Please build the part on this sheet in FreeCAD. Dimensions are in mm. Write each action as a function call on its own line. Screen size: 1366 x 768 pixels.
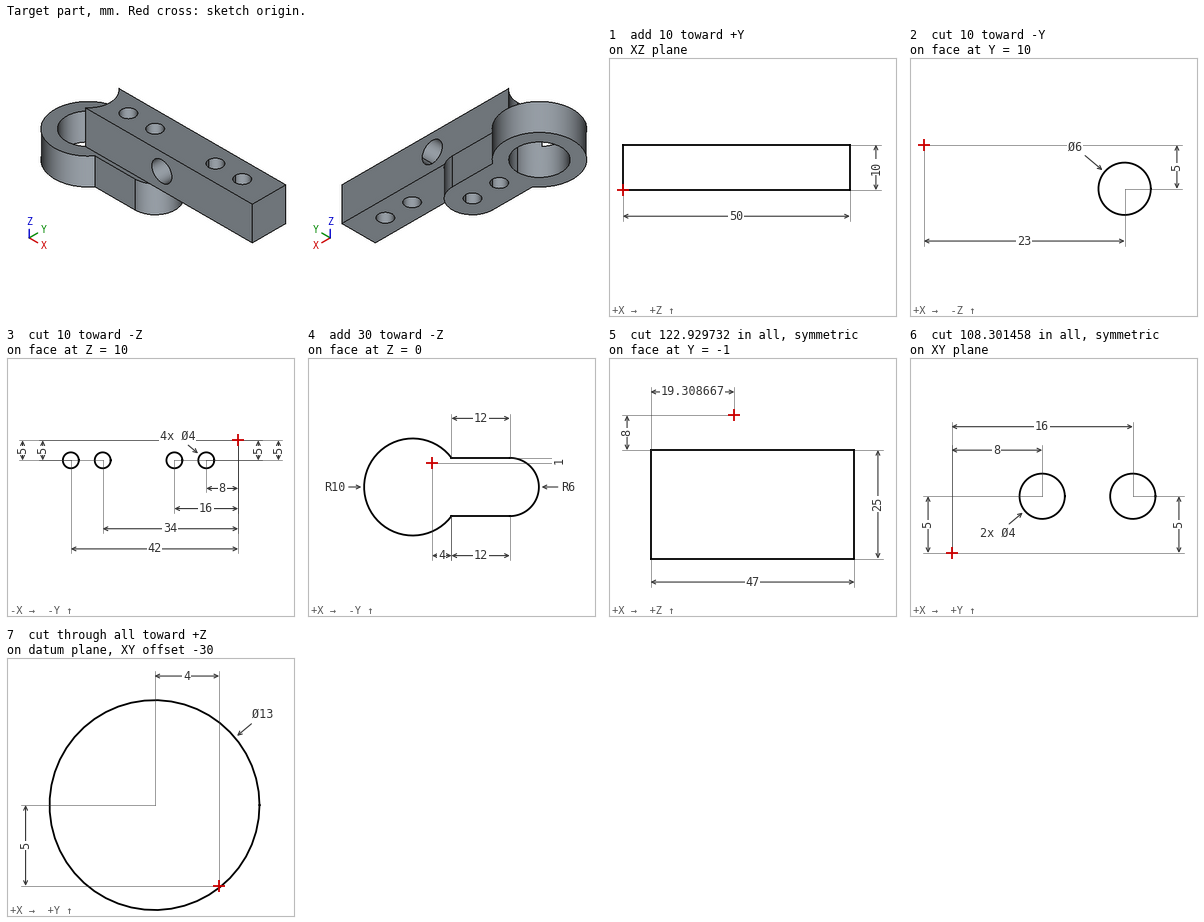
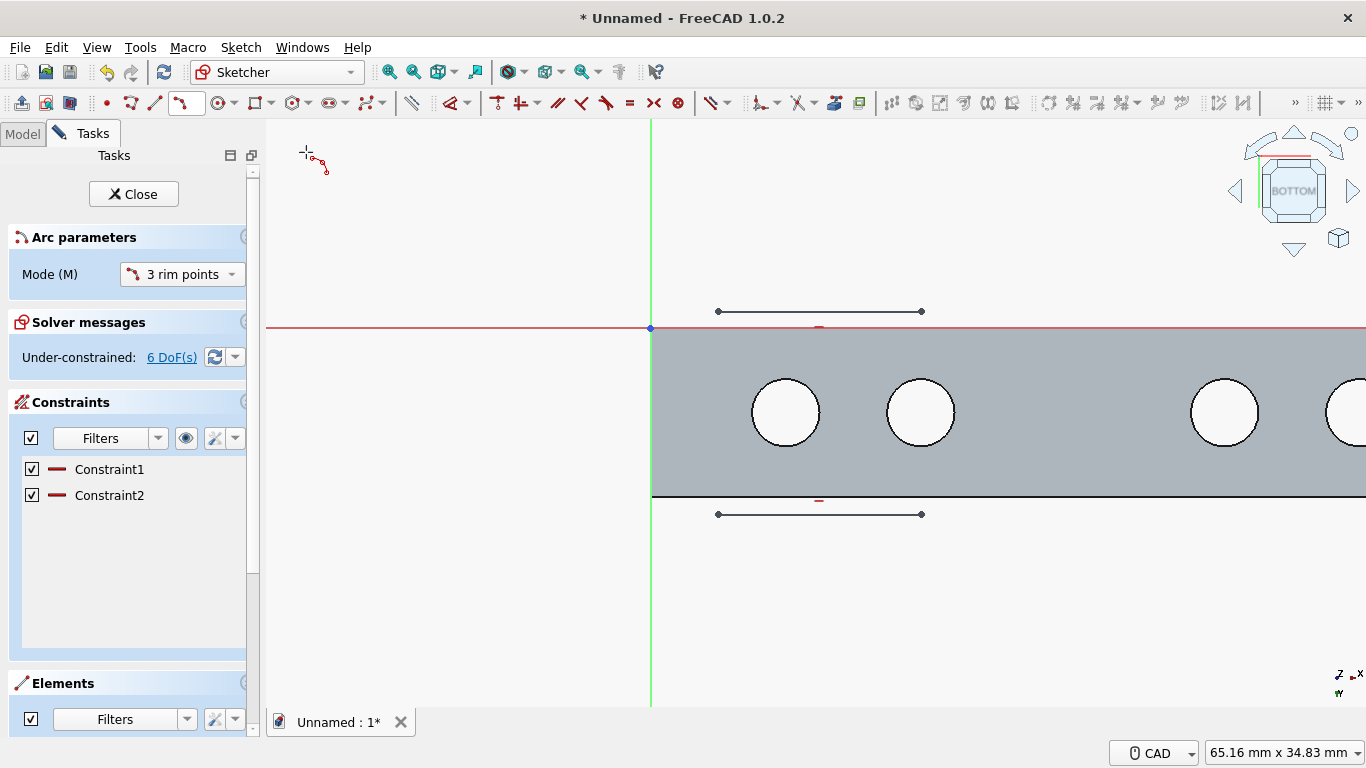
click(921, 515)
click(921, 312)
click(1022, 413)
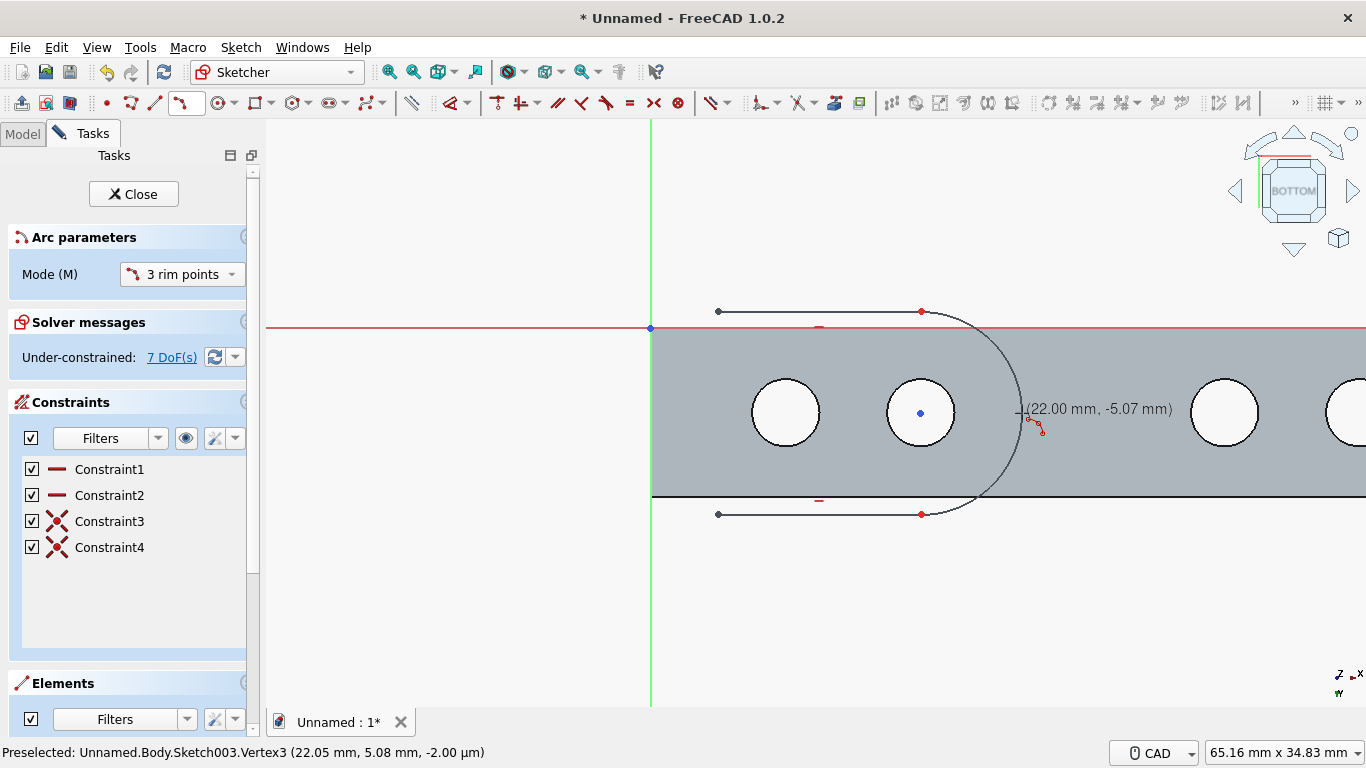
click(718, 312)
click(718, 515)
click(414, 413)
key(Escape)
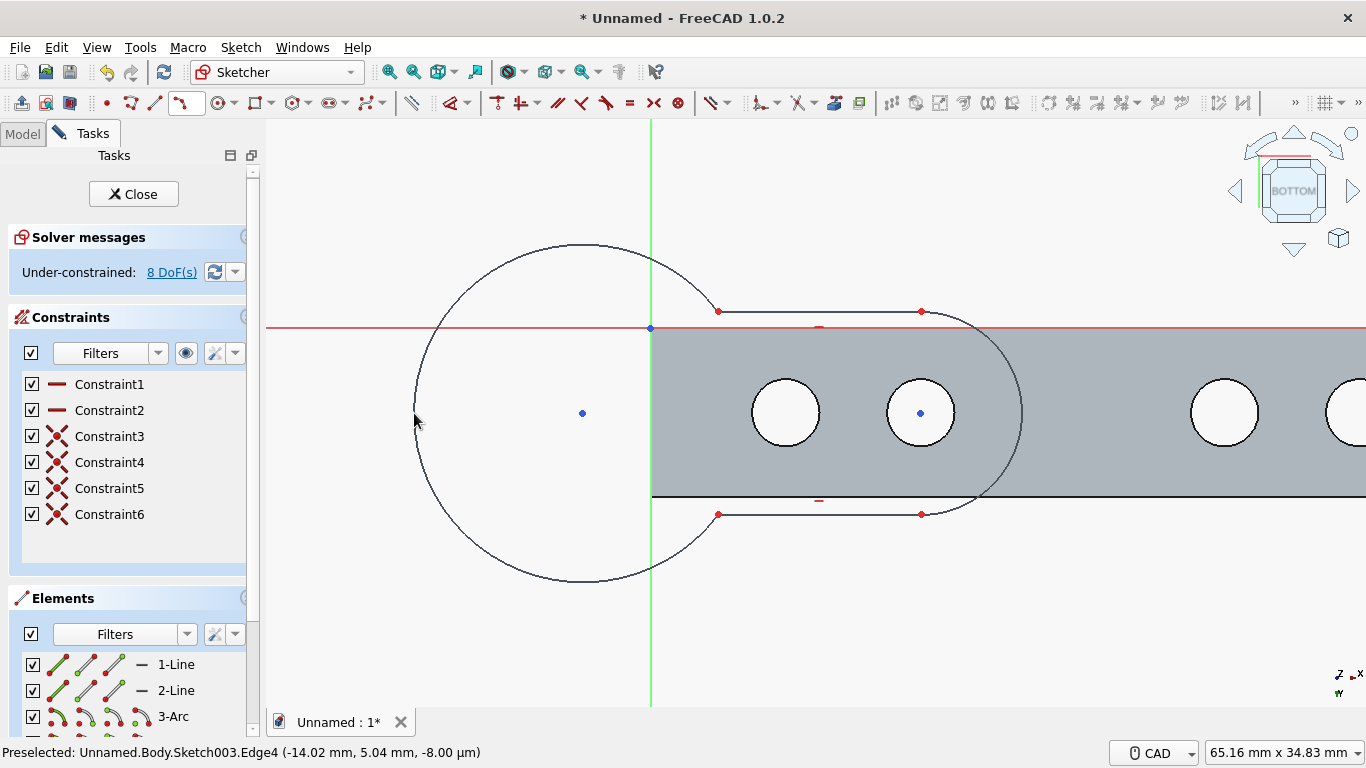
click(779, 515)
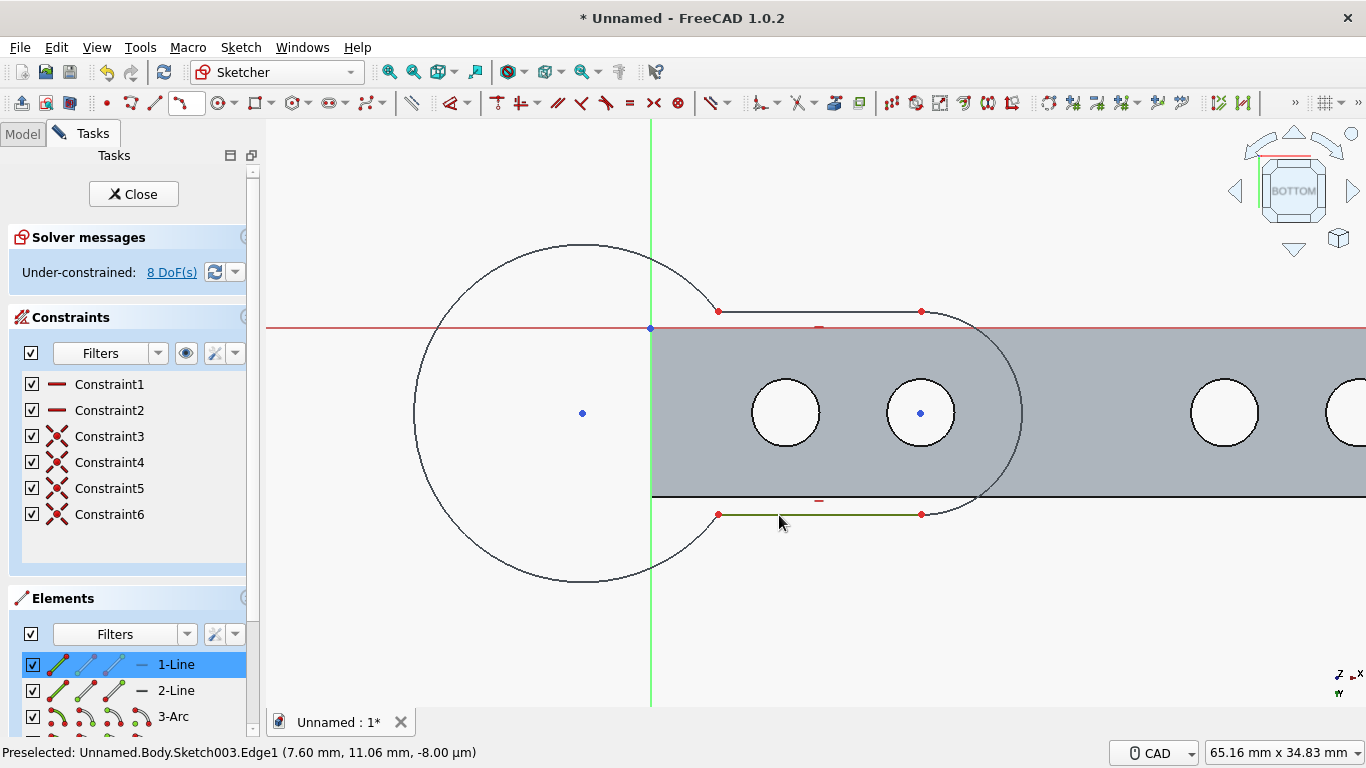
click(1003, 473)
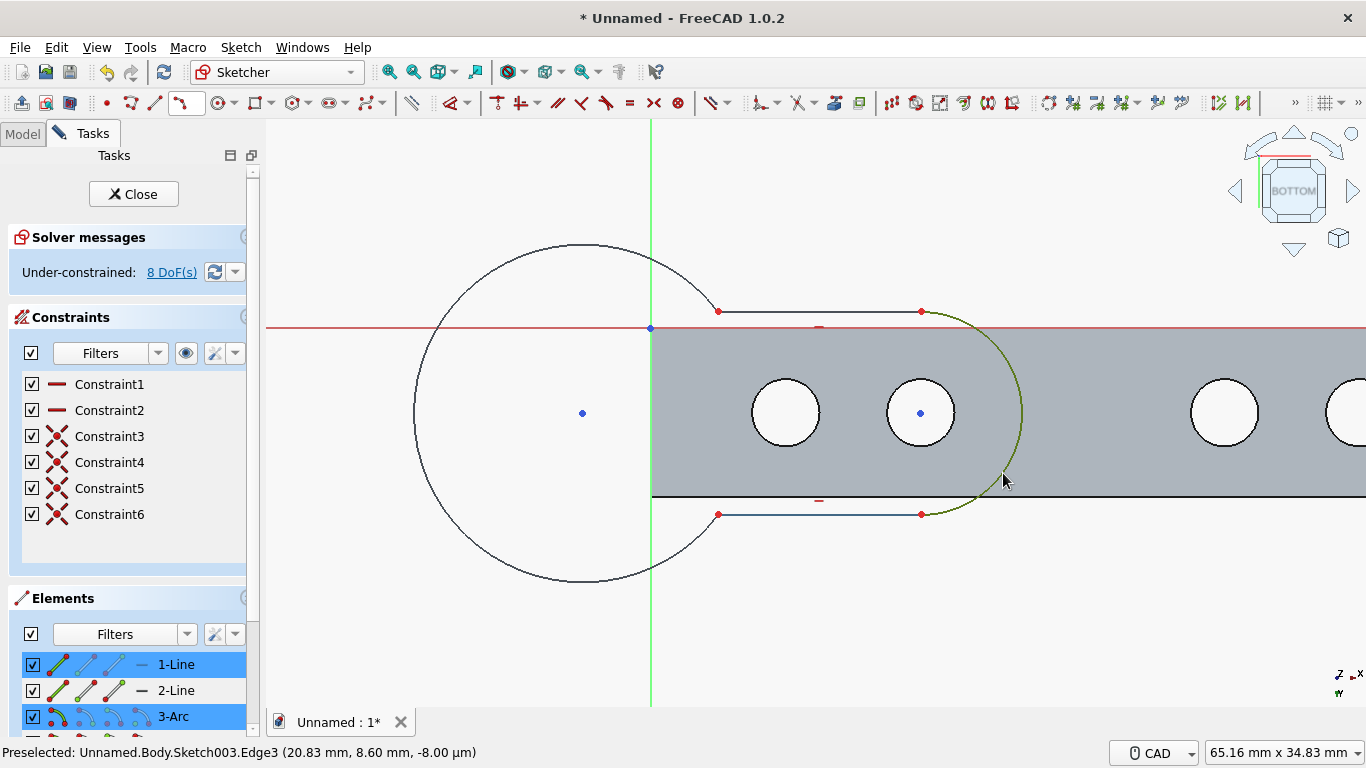
click(606, 104)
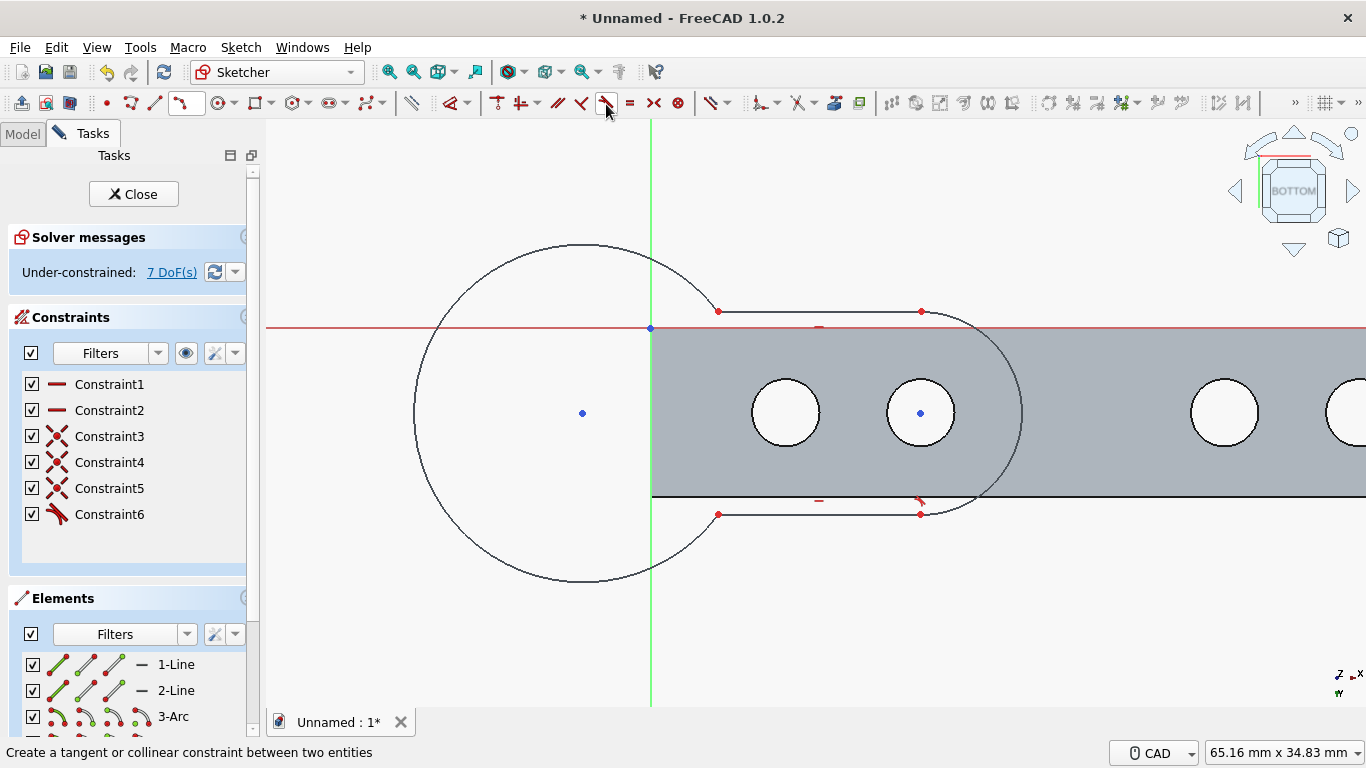
click(860, 312)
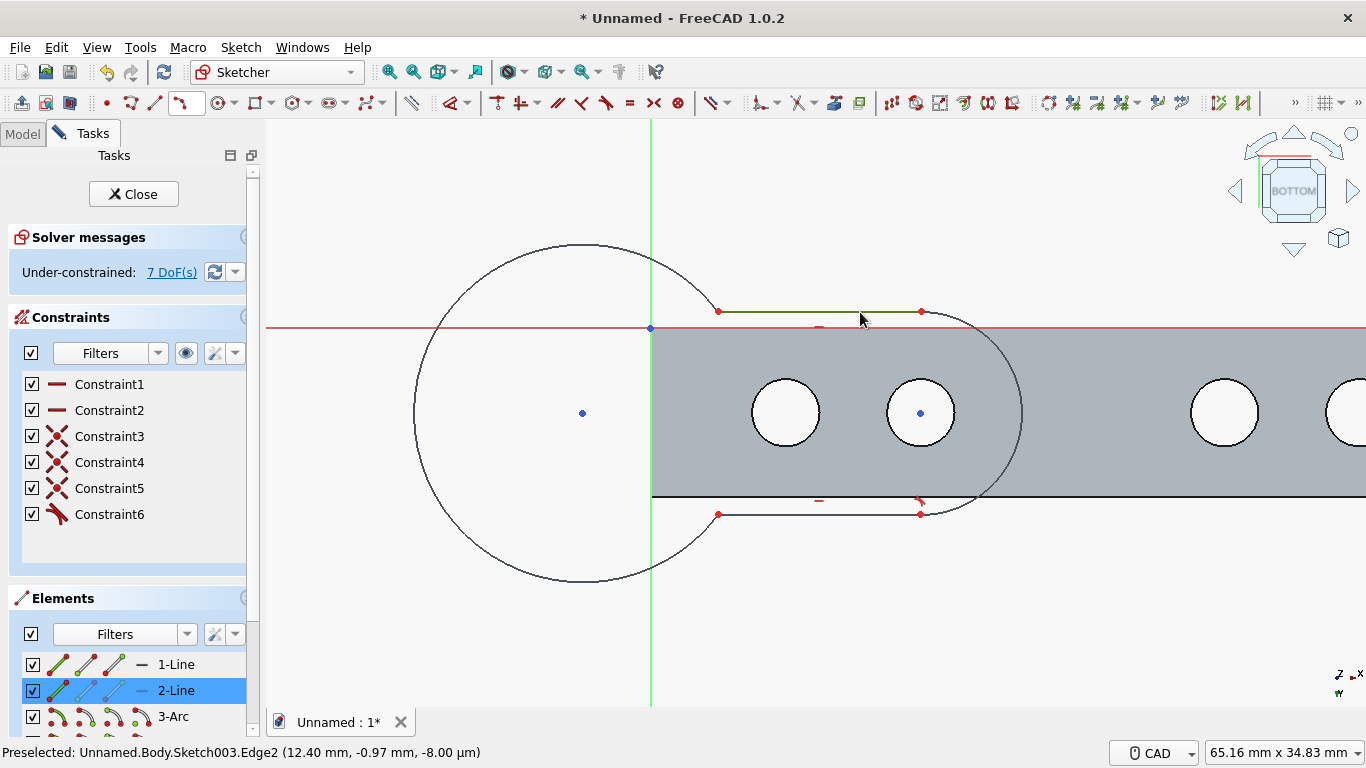
click(1003, 473)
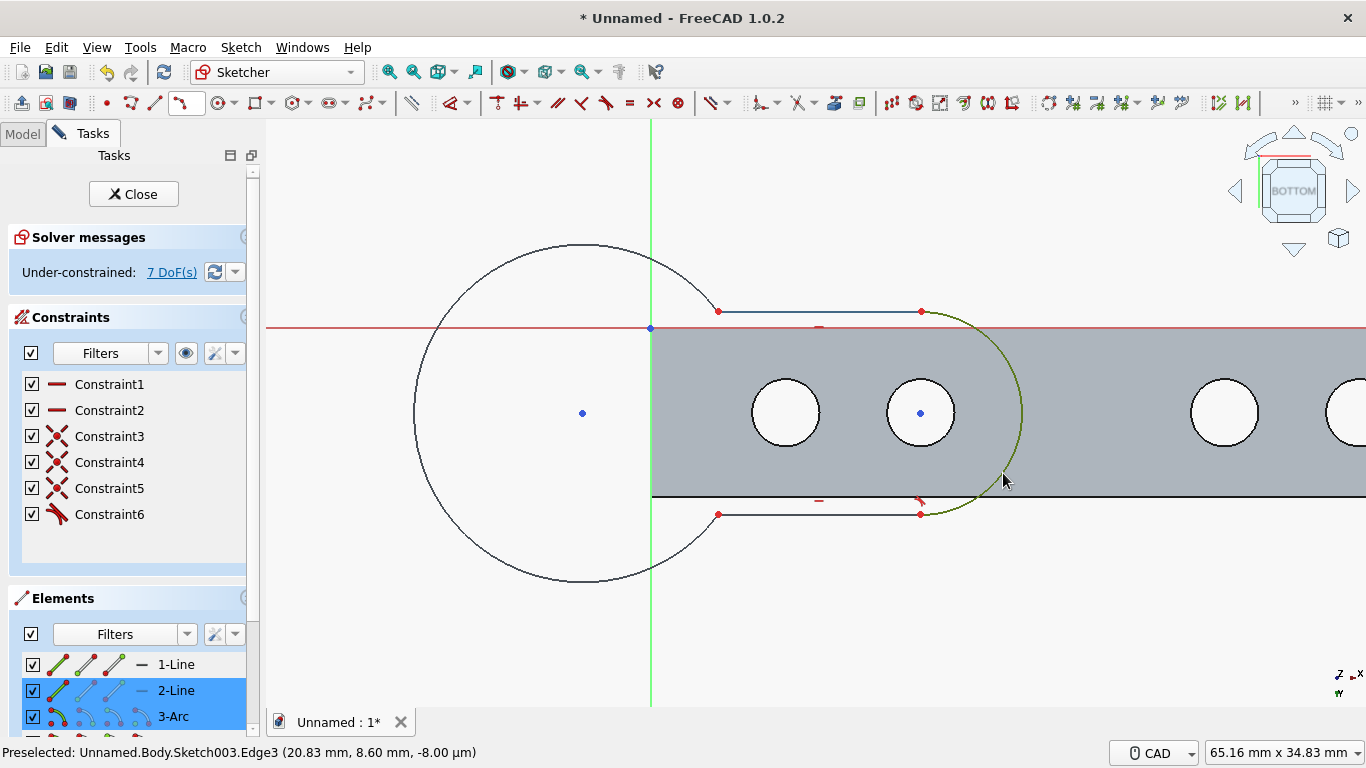
click(606, 104)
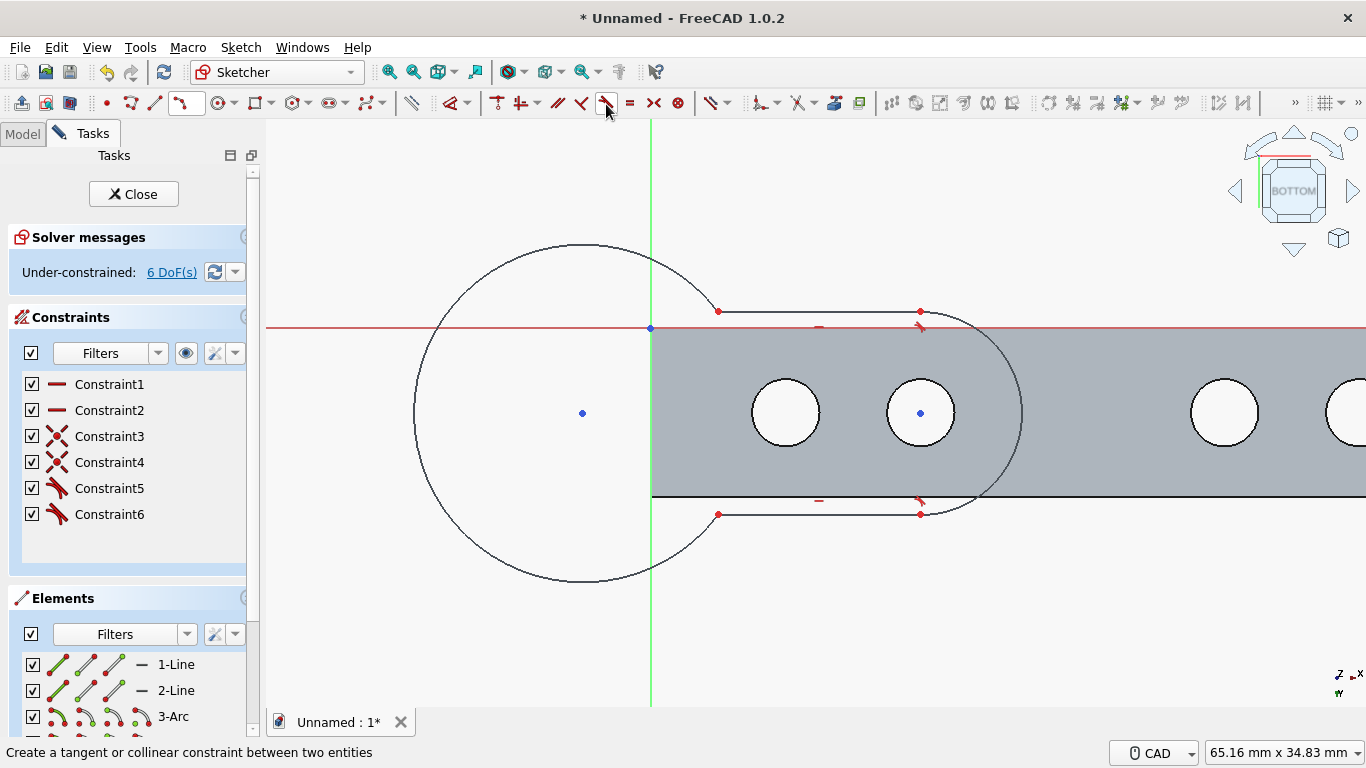
click(450, 104)